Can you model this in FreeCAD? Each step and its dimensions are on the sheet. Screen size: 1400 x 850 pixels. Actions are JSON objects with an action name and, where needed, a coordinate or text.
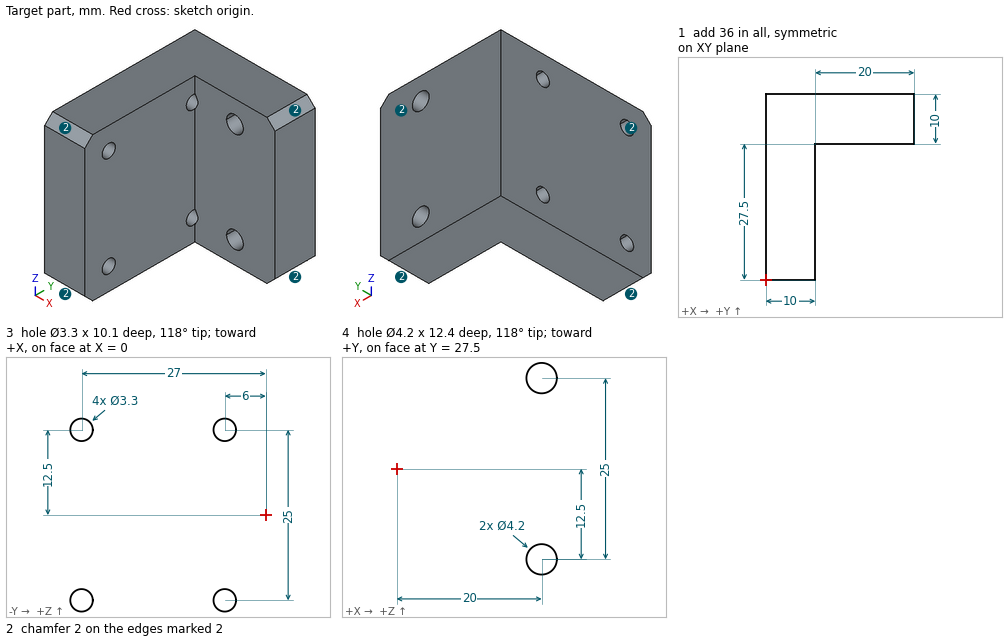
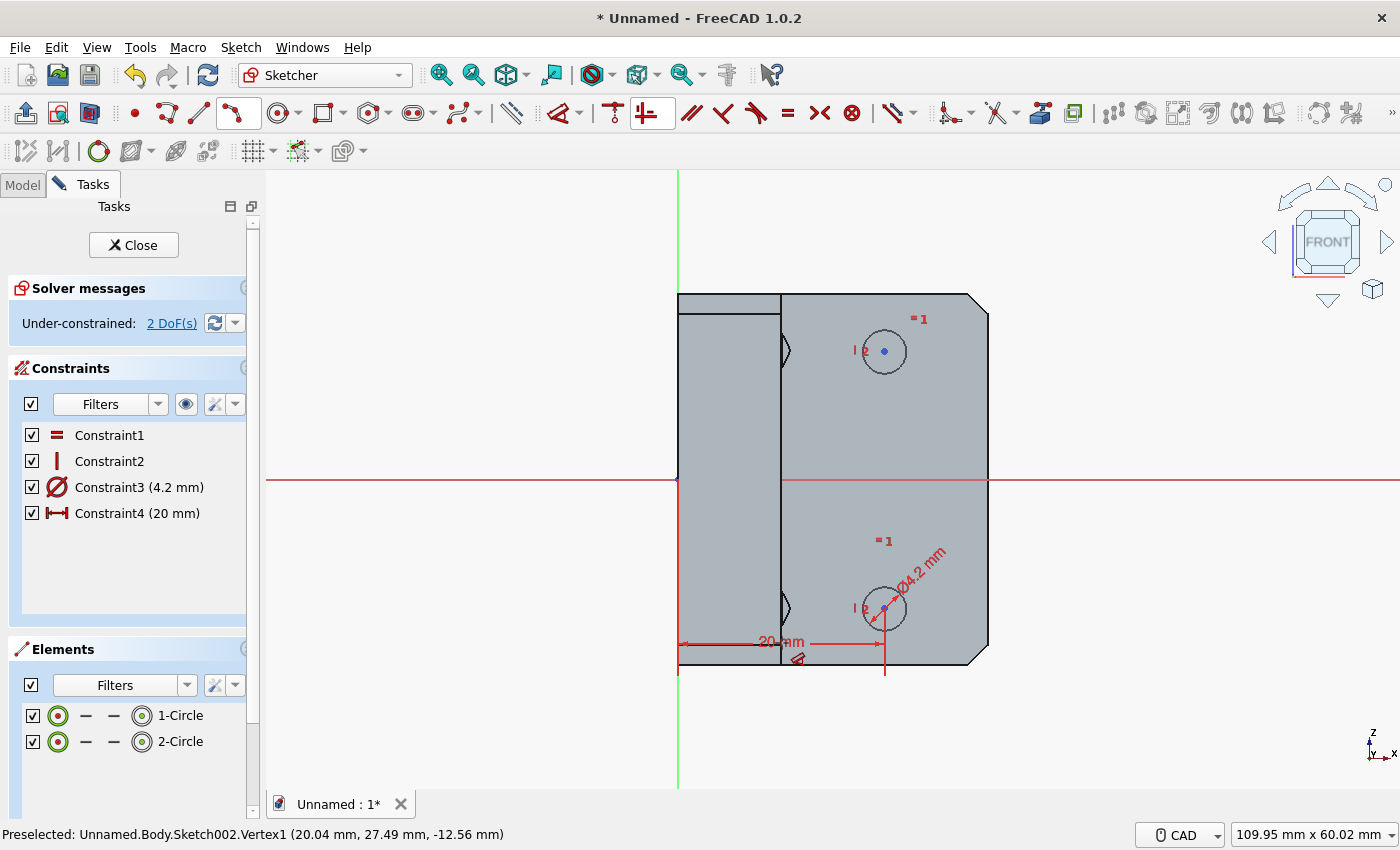
{"action": "left_click", "coordinate": [885, 609]}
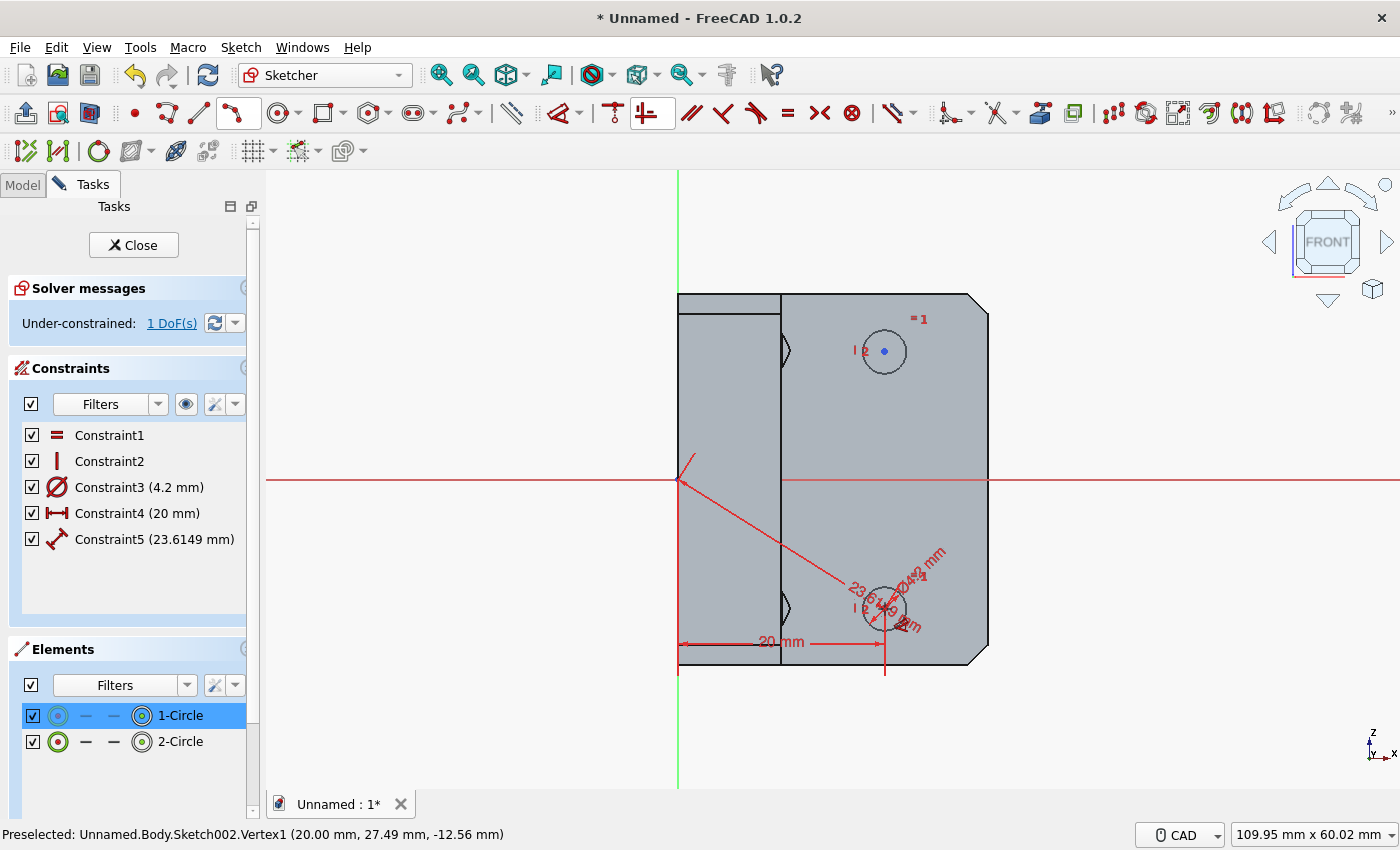
{"action": "left_click", "coordinate": [885, 352]}
{"action": "left_click", "coordinate": [919, 421]}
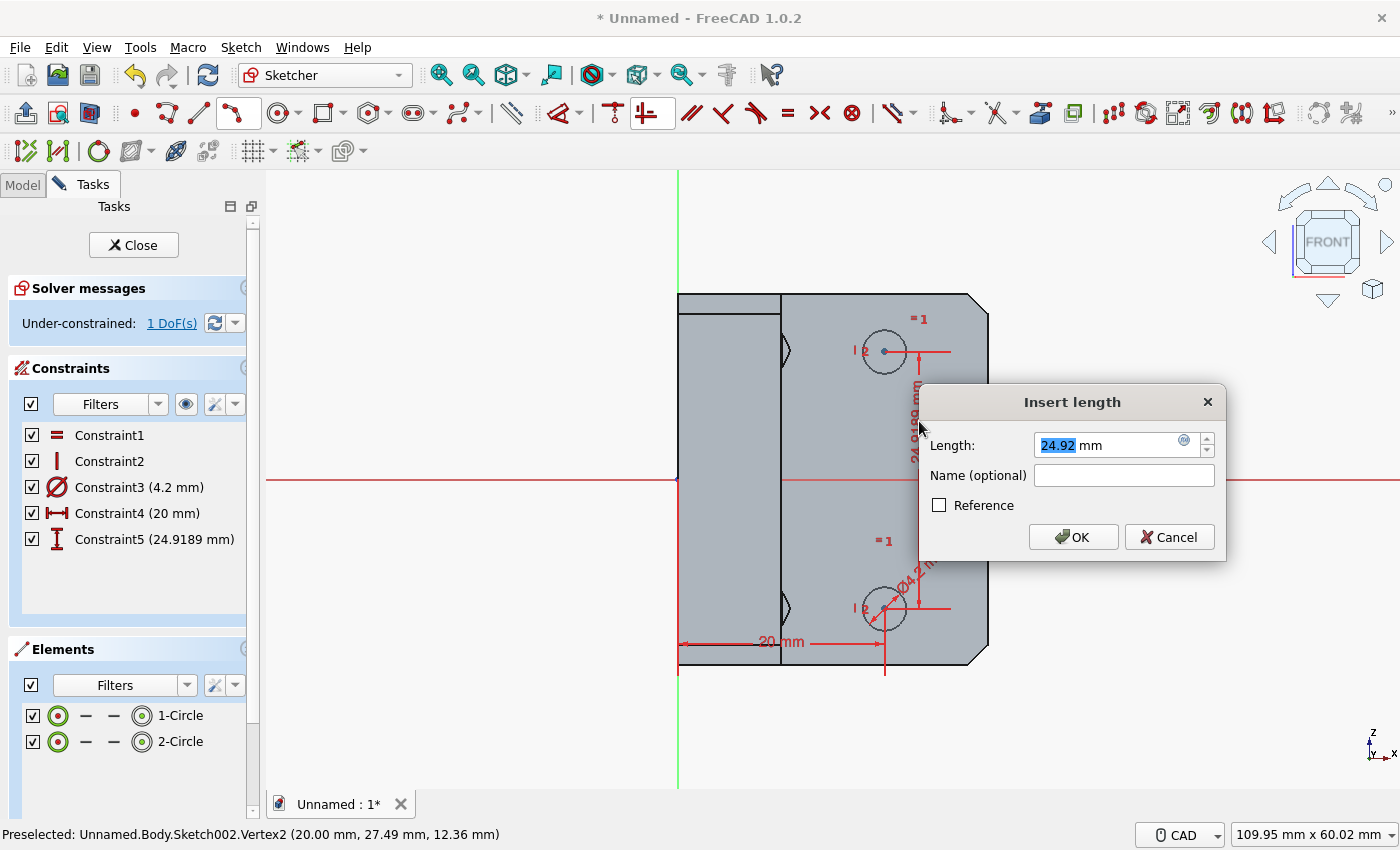
{"action": "type", "text": "25"}
{"action": "key", "text": "Return"}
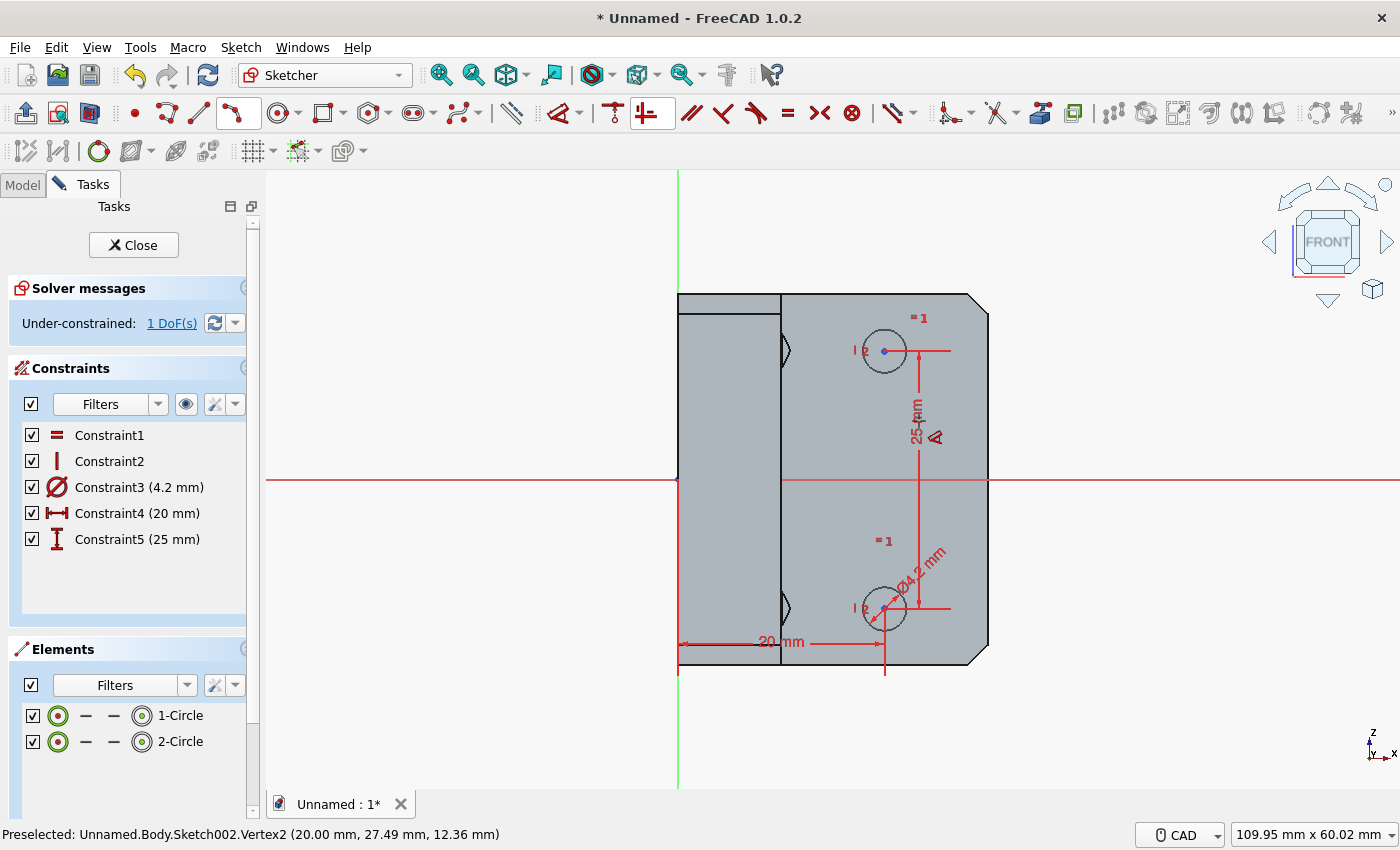
{"action": "left_click", "coordinate": [885, 609]}
{"action": "left_click", "coordinate": [644, 544]}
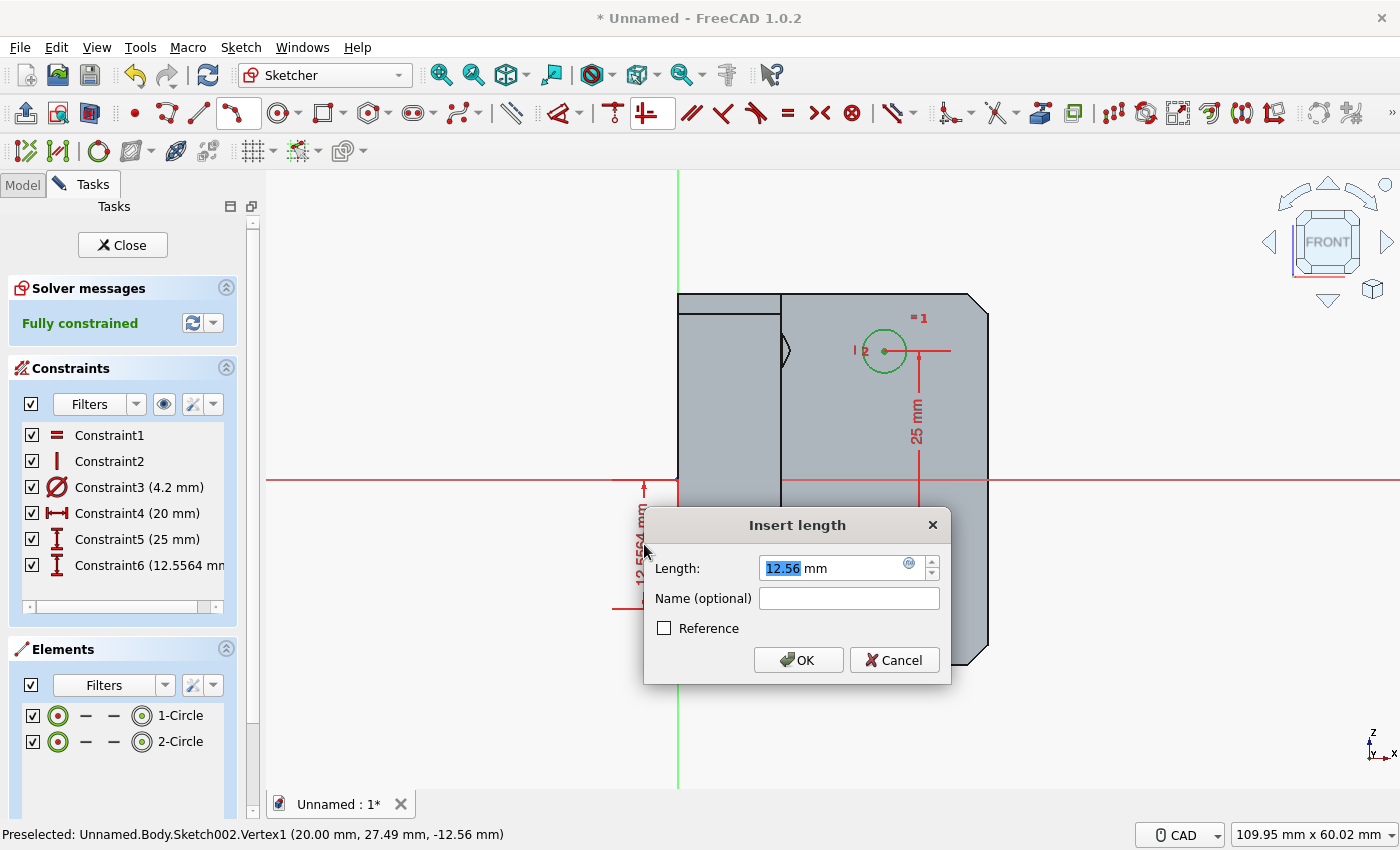
{"action": "type", "text": "12.5"}
{"action": "key", "text": "Return"}
{"action": "key", "text": "Escape"}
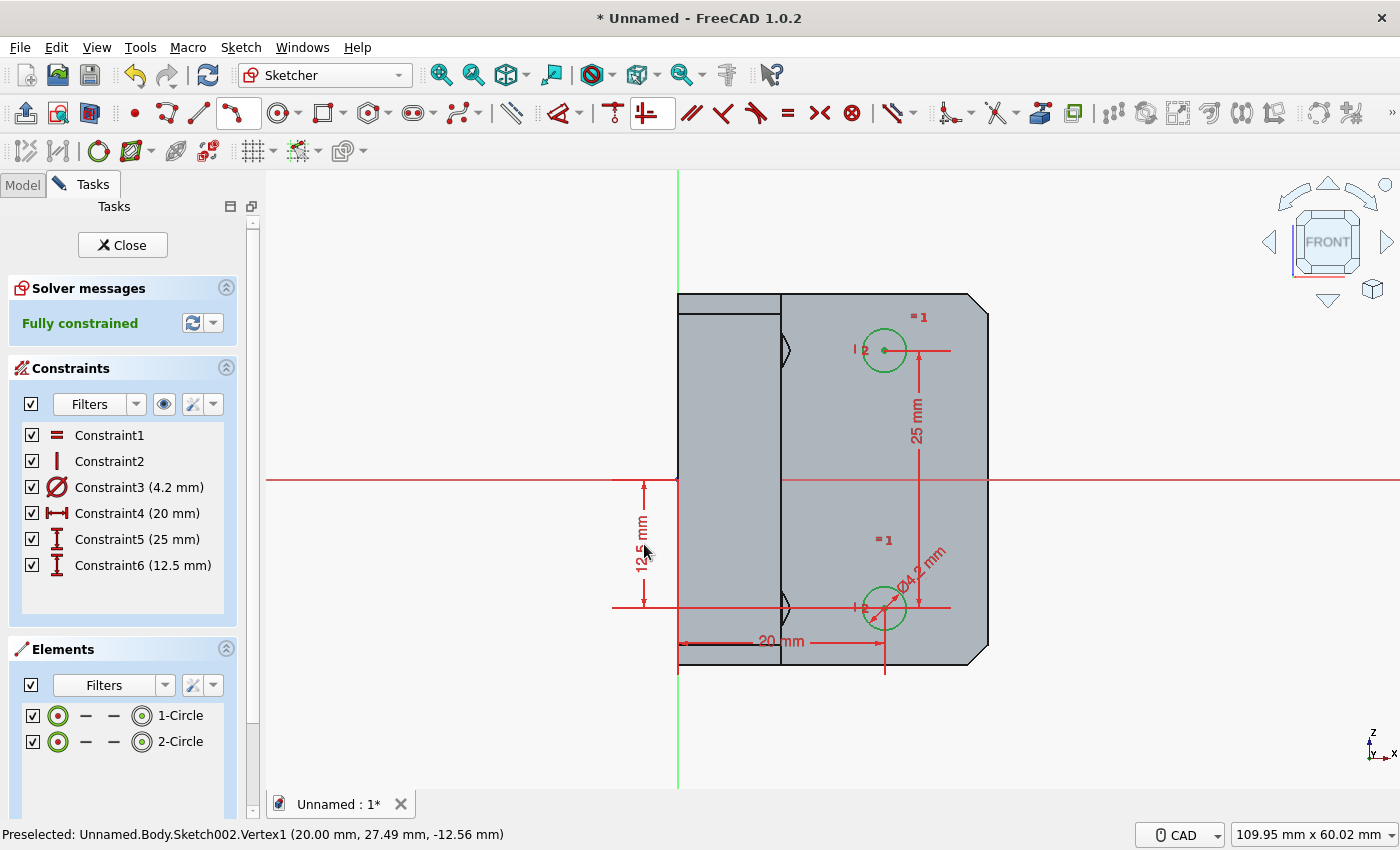
{"action": "left_click", "coordinate": [123, 245]}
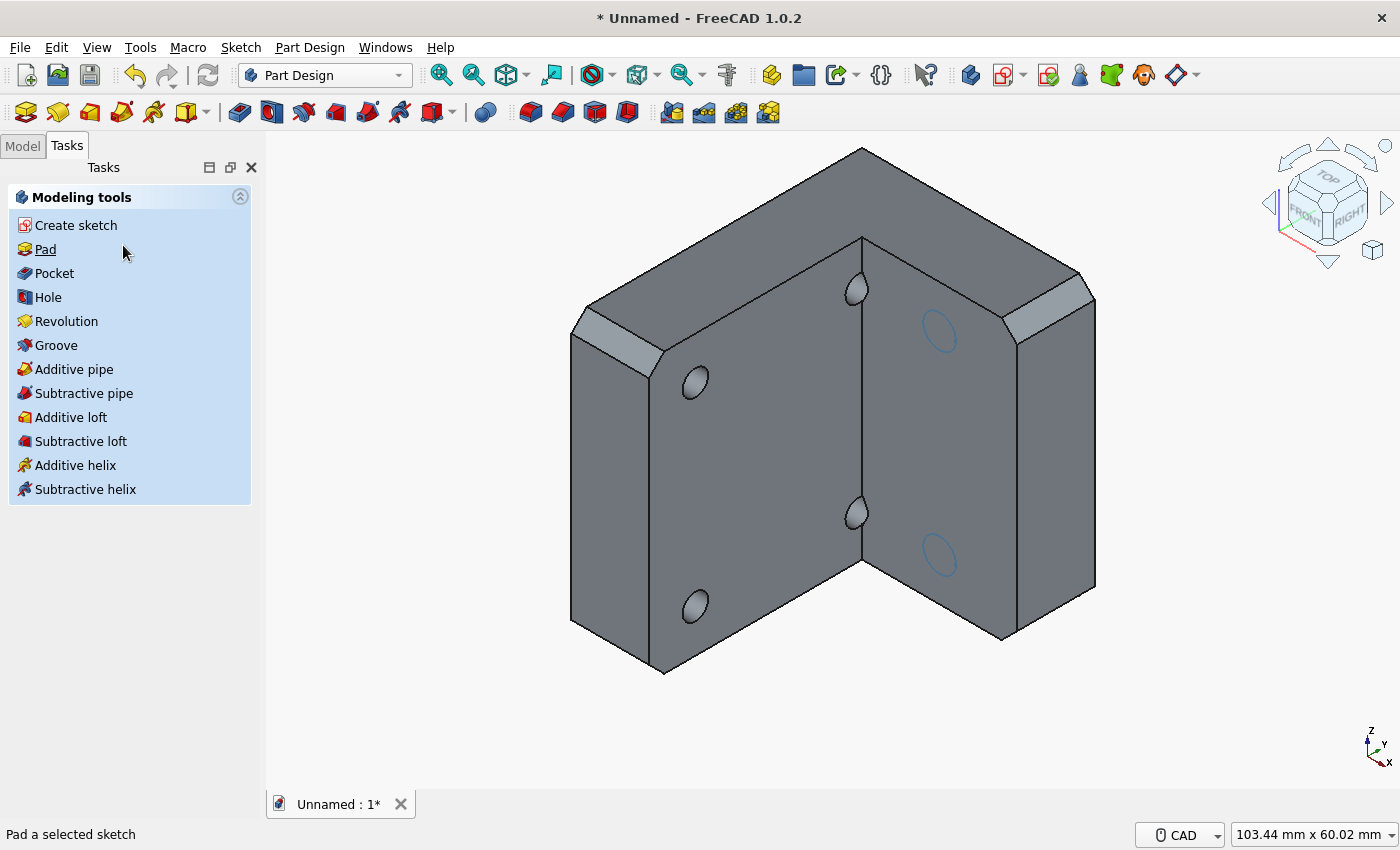
{"action": "left_click", "coordinate": [272, 112]}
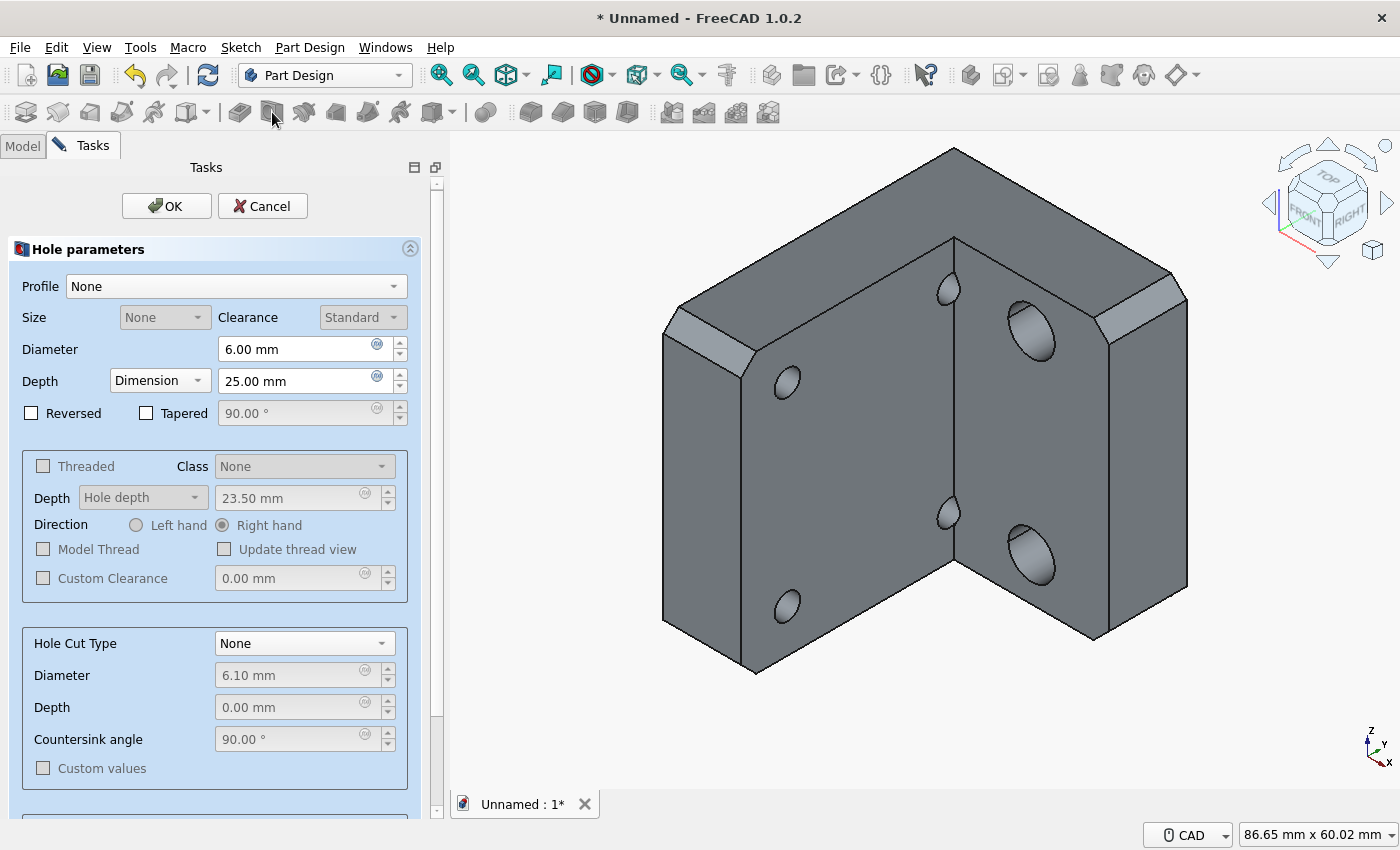
{"action": "triple_click", "coordinate": [305, 349]}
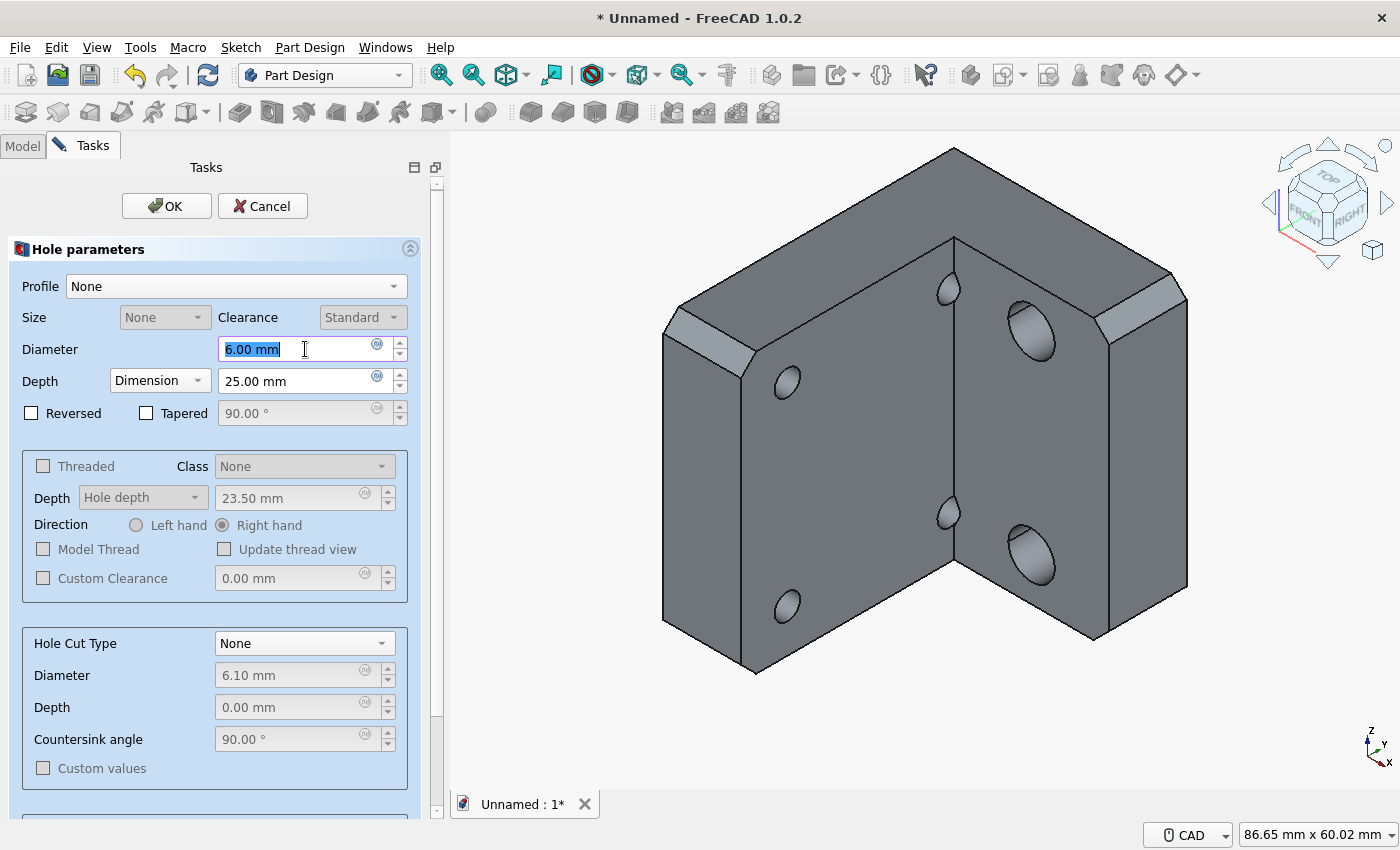
{"action": "type", "text": "4.2"}
{"action": "key", "text": "Tab"}